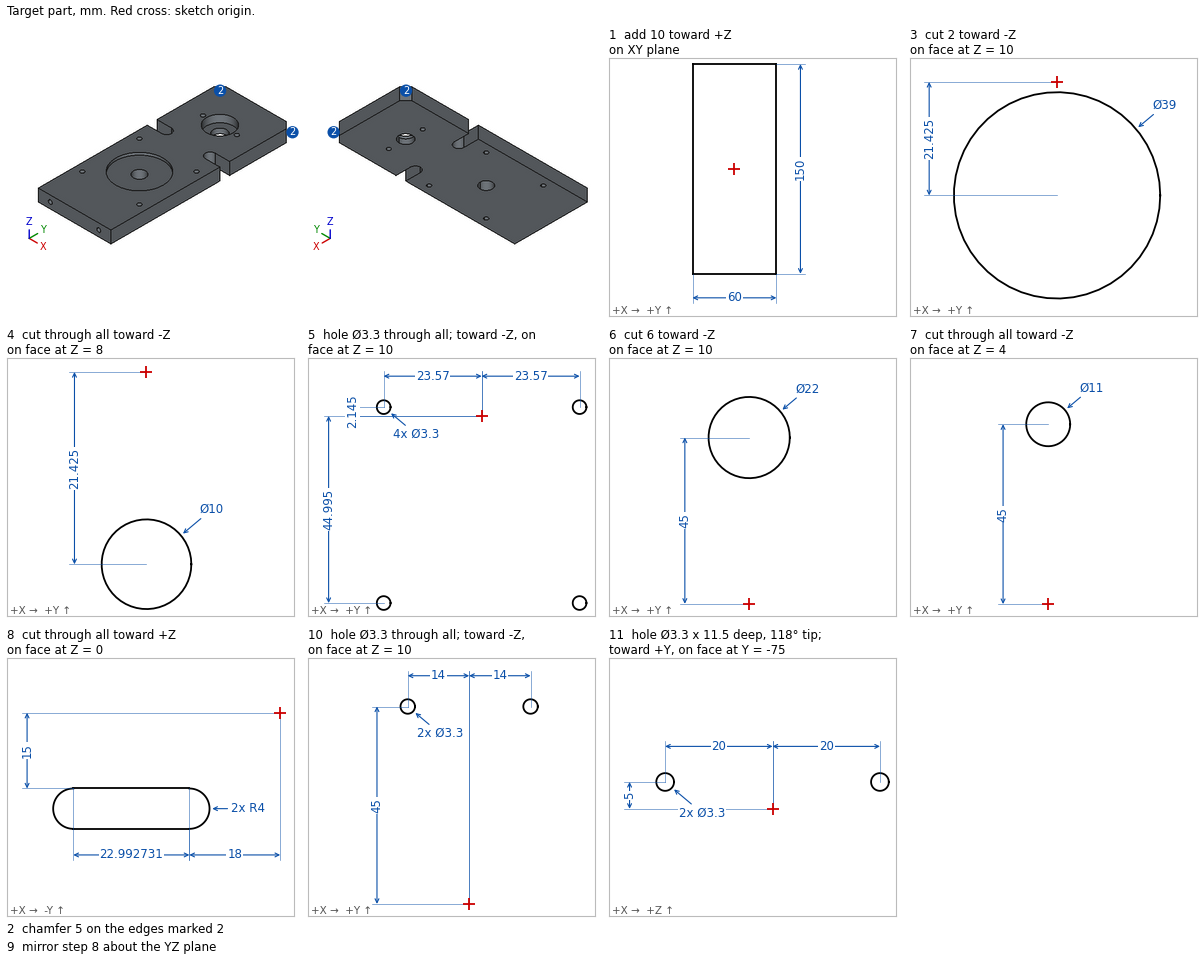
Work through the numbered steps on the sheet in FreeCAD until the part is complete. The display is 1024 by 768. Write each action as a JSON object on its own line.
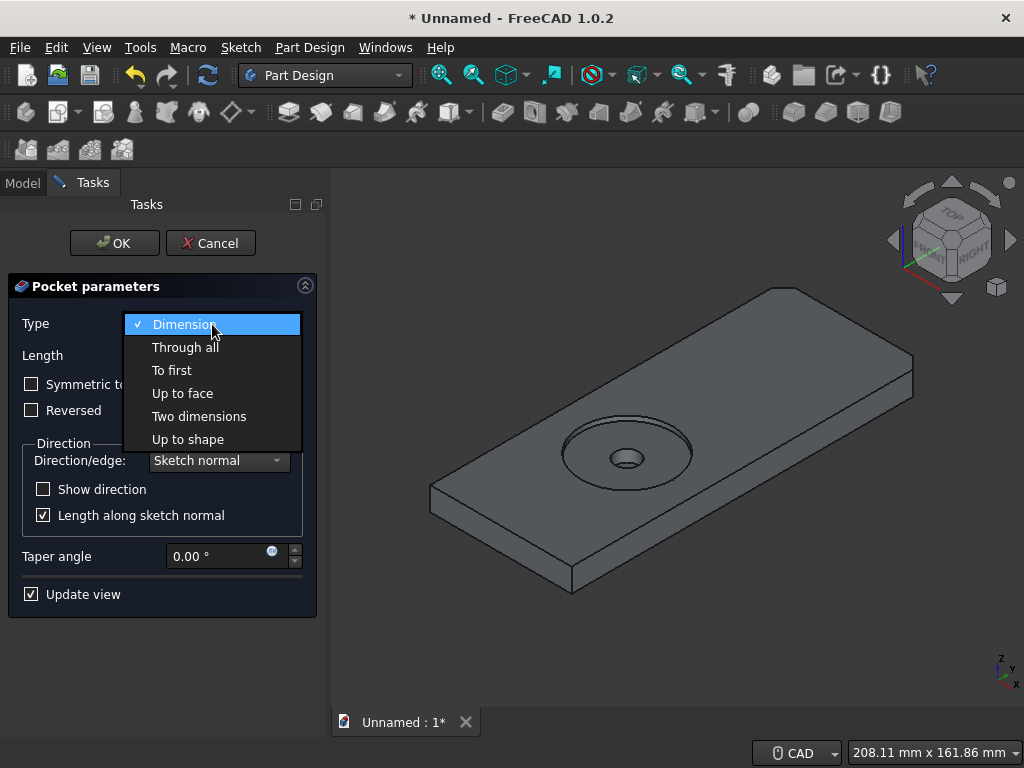
{"action": "left_click", "coordinate": [212, 348]}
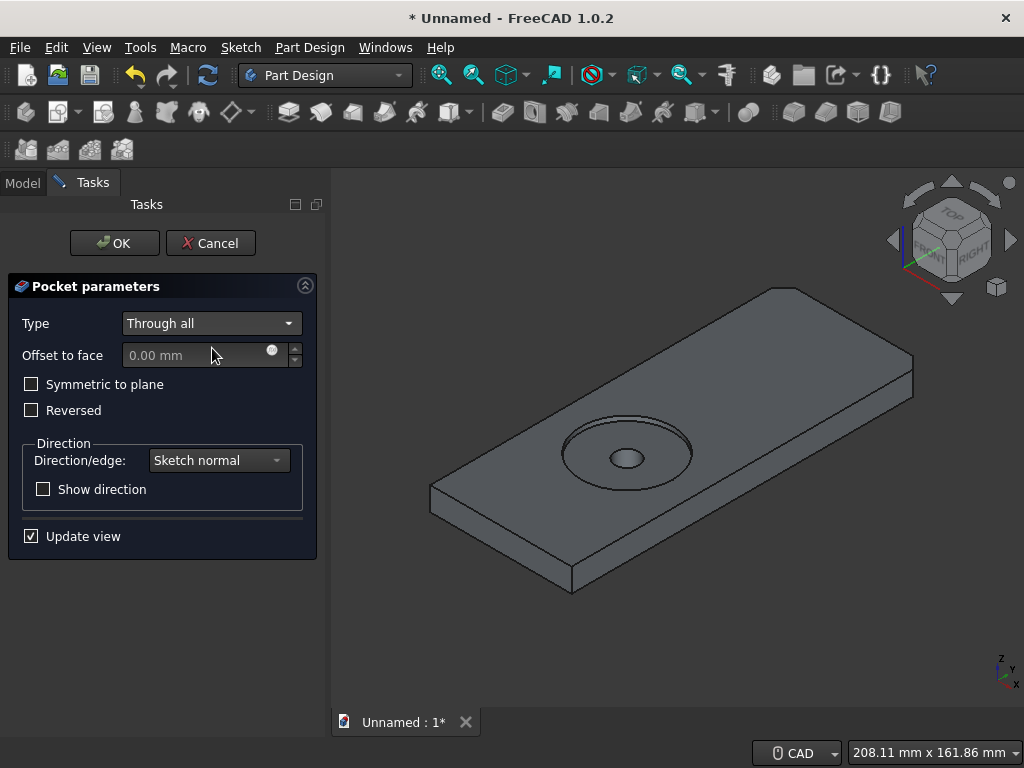
{"action": "left_click", "coordinate": [115, 243]}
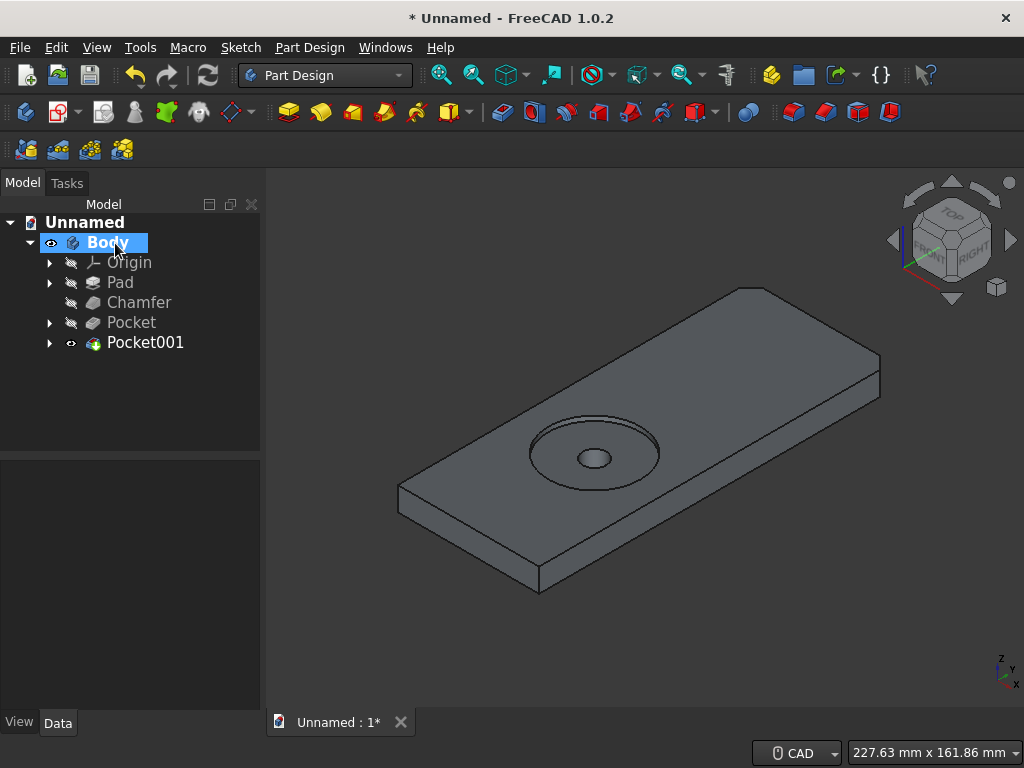
{"action": "left_click", "coordinate": [746, 365]}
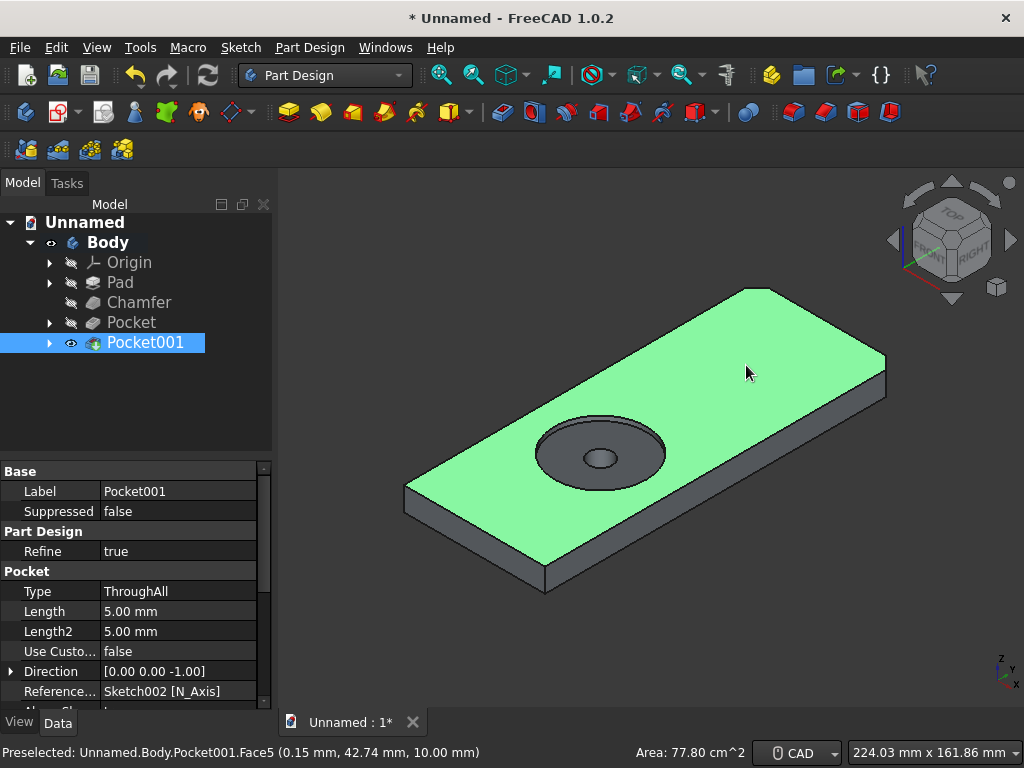
{"action": "left_click", "coordinate": [58, 112]}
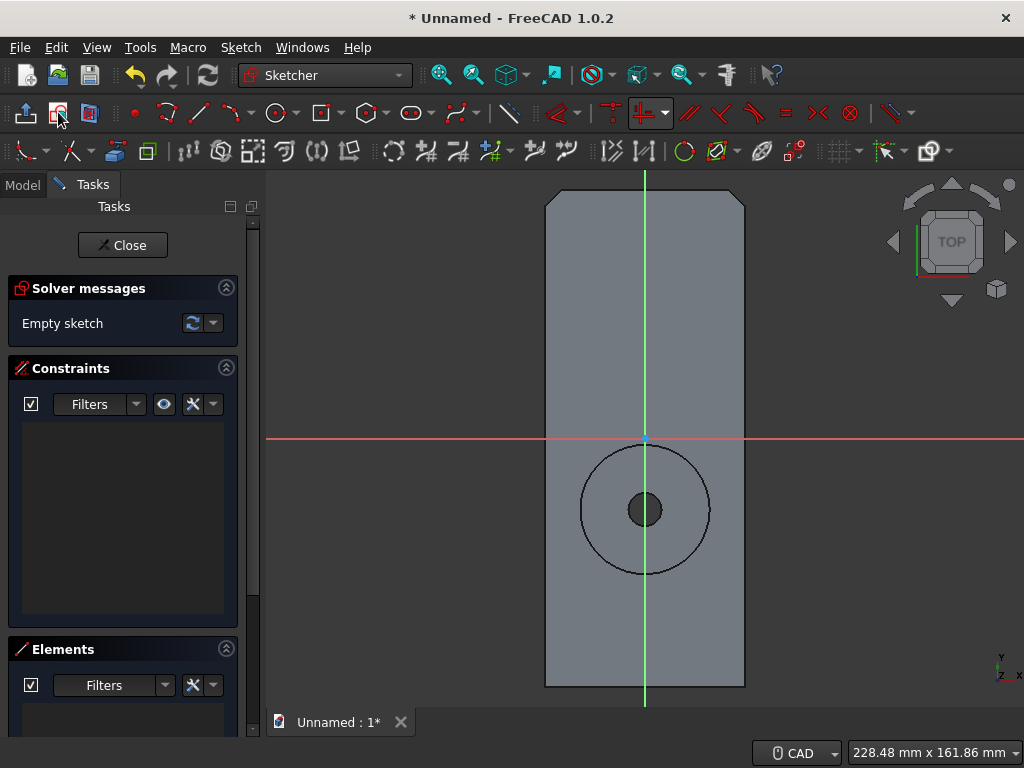
{"action": "scroll", "coordinate": [701, 568], "scroll_direction": "up", "scroll_amount": 4}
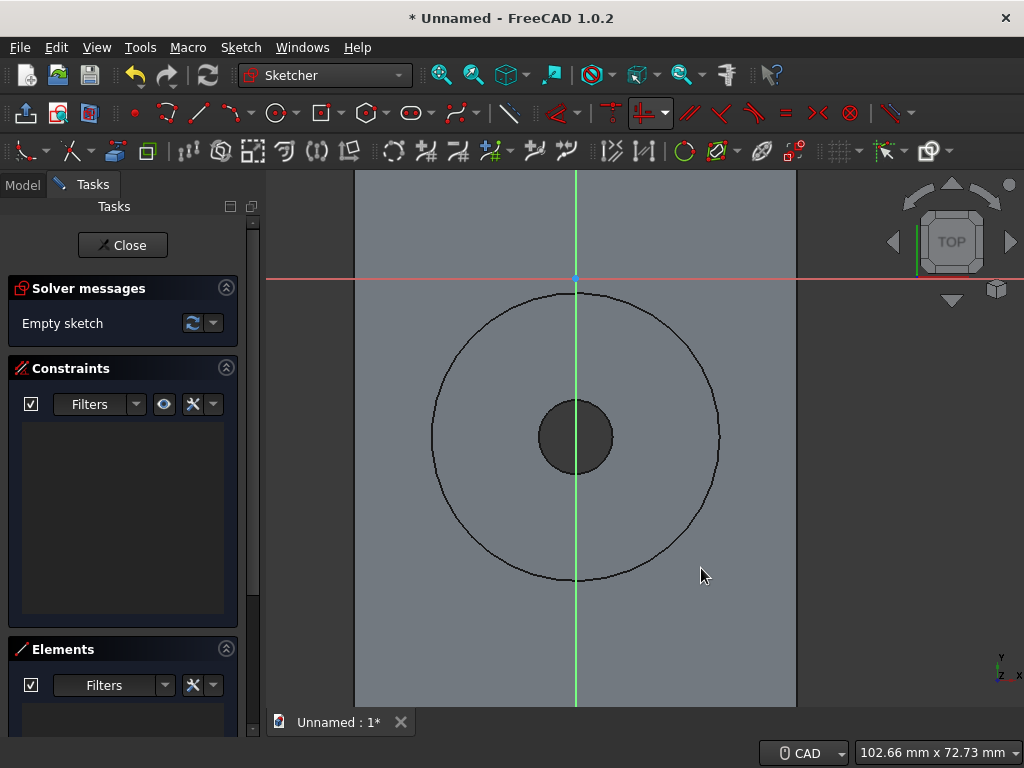
{"action": "left_click", "coordinate": [276, 114]}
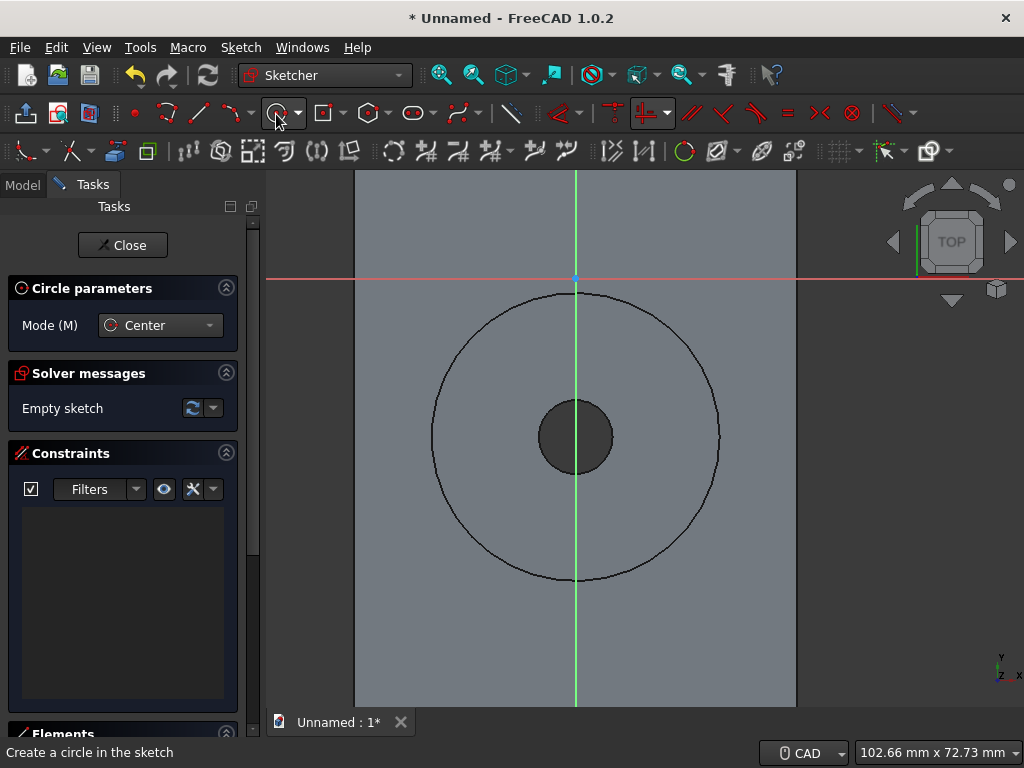
{"action": "scroll", "coordinate": [402, 263], "scroll_direction": "up", "scroll_amount": 4}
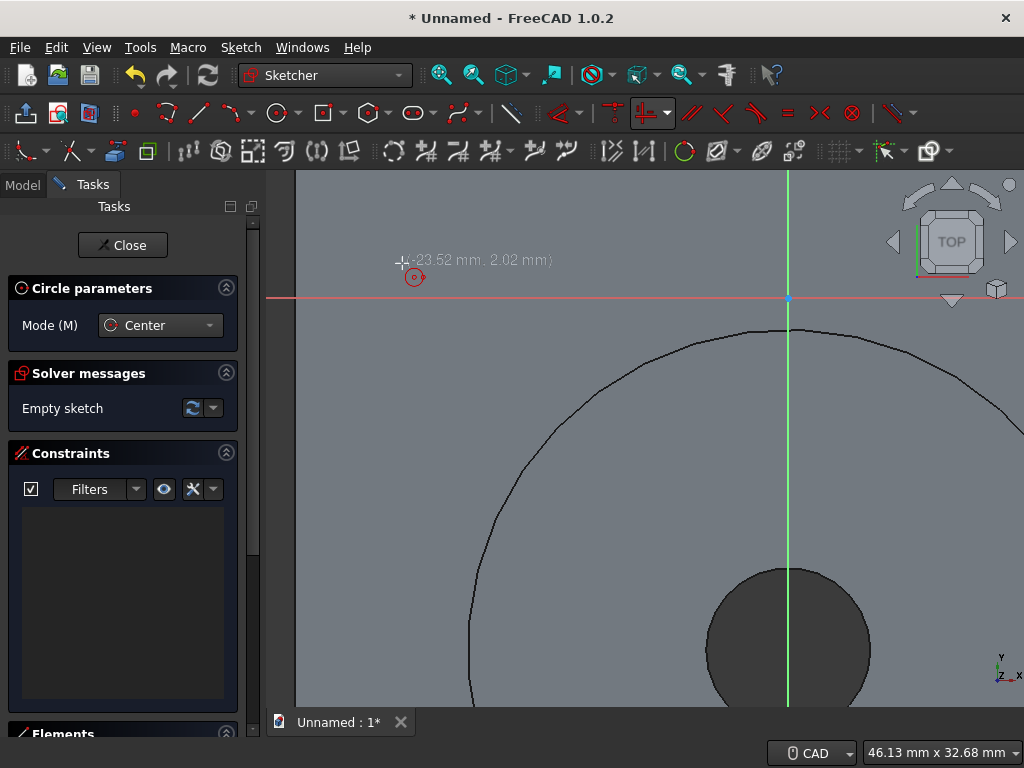
{"action": "left_click", "coordinate": [401, 263]}
{"action": "left_click", "coordinate": [420, 244]}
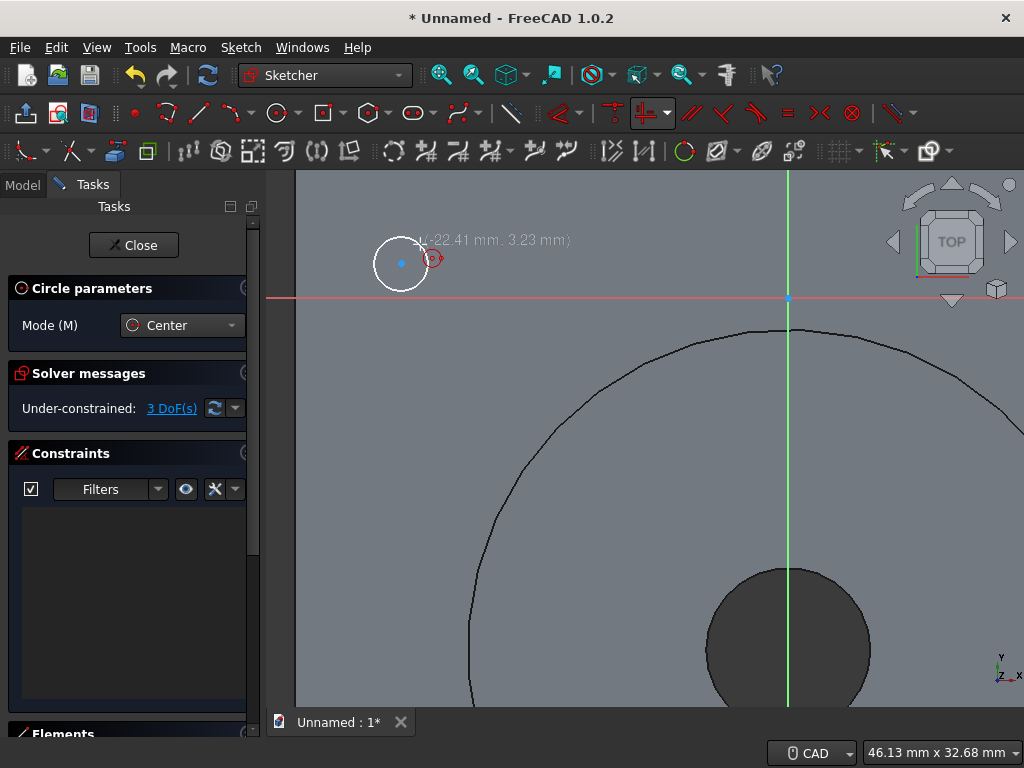
{"action": "scroll", "coordinate": [404, 266], "scroll_direction": "down", "scroll_amount": 4}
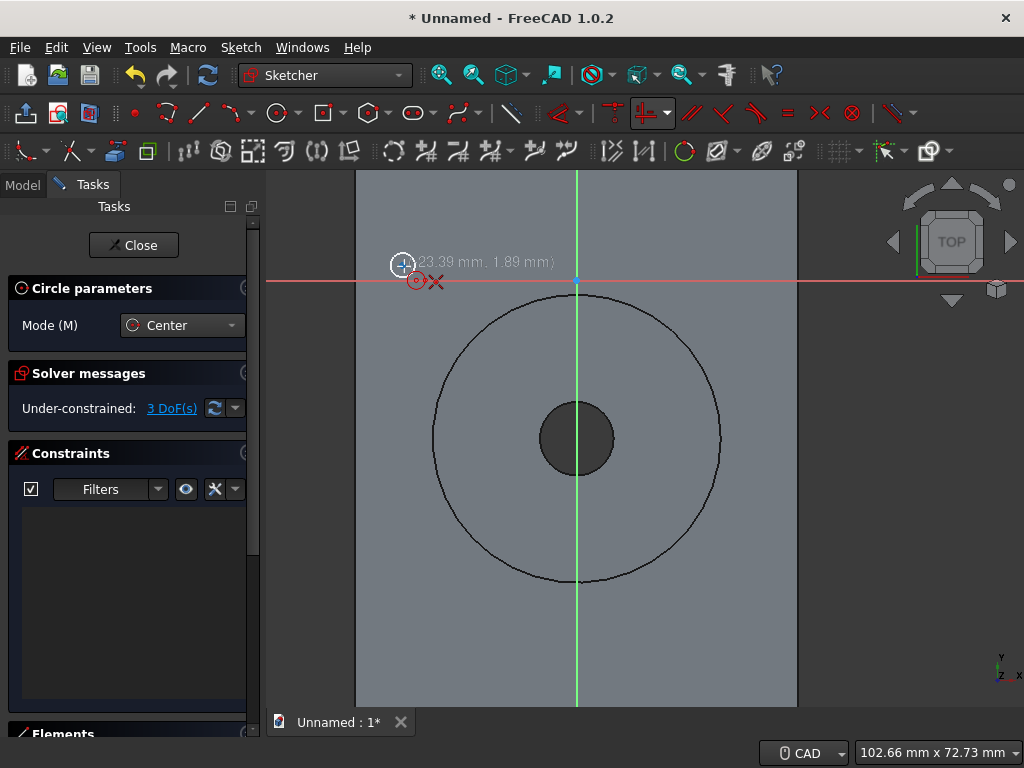
{"action": "scroll", "coordinate": [403, 613], "scroll_direction": "up", "scroll_amount": 4}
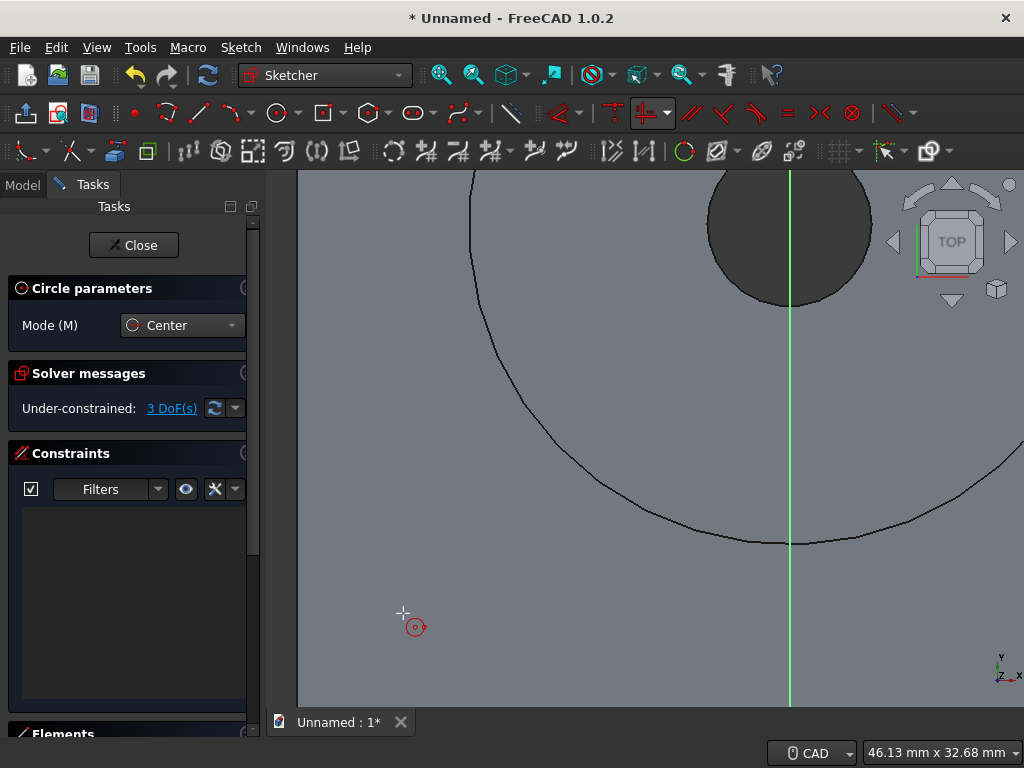
{"action": "left_click", "coordinate": [402, 611]}
{"action": "left_click", "coordinate": [421, 592]}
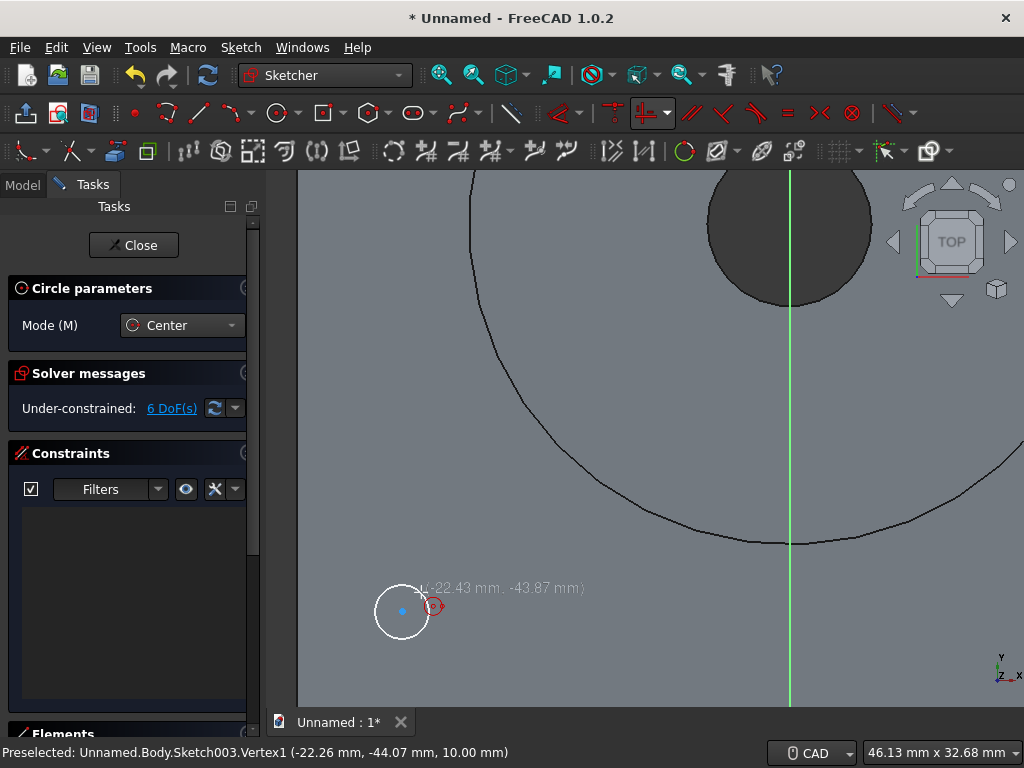
{"action": "scroll", "coordinate": [403, 613], "scroll_direction": "down", "scroll_amount": 4}